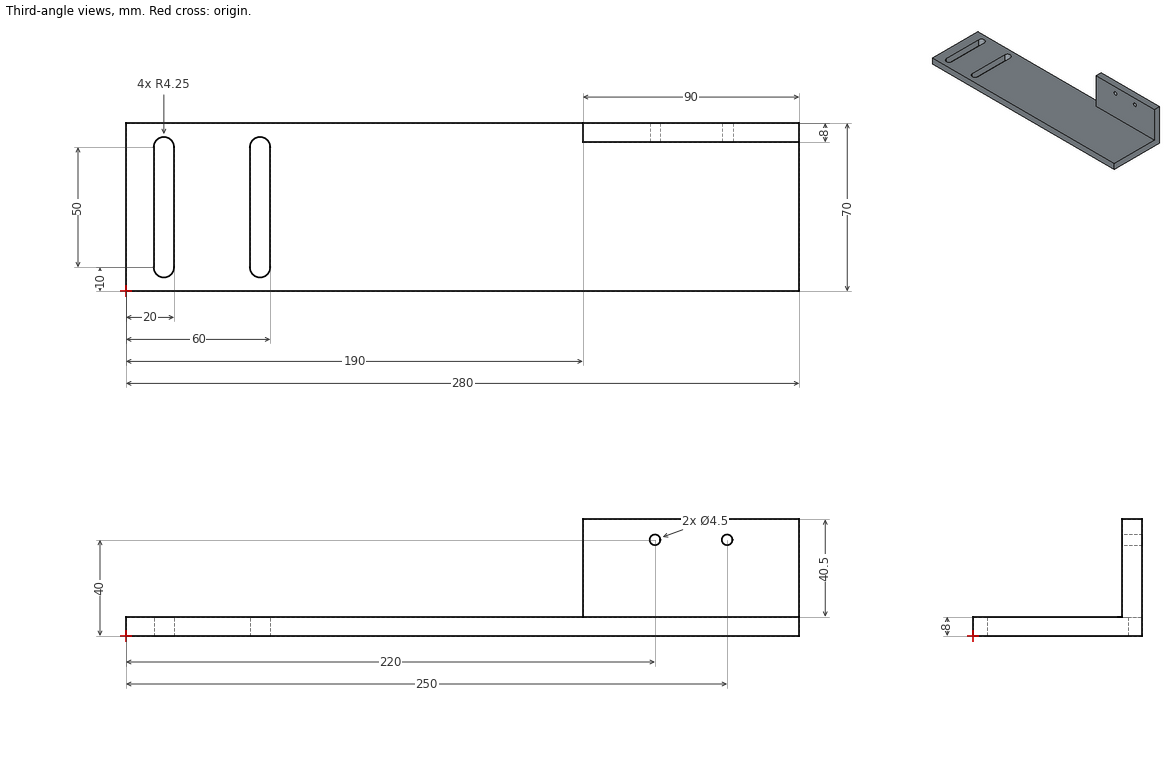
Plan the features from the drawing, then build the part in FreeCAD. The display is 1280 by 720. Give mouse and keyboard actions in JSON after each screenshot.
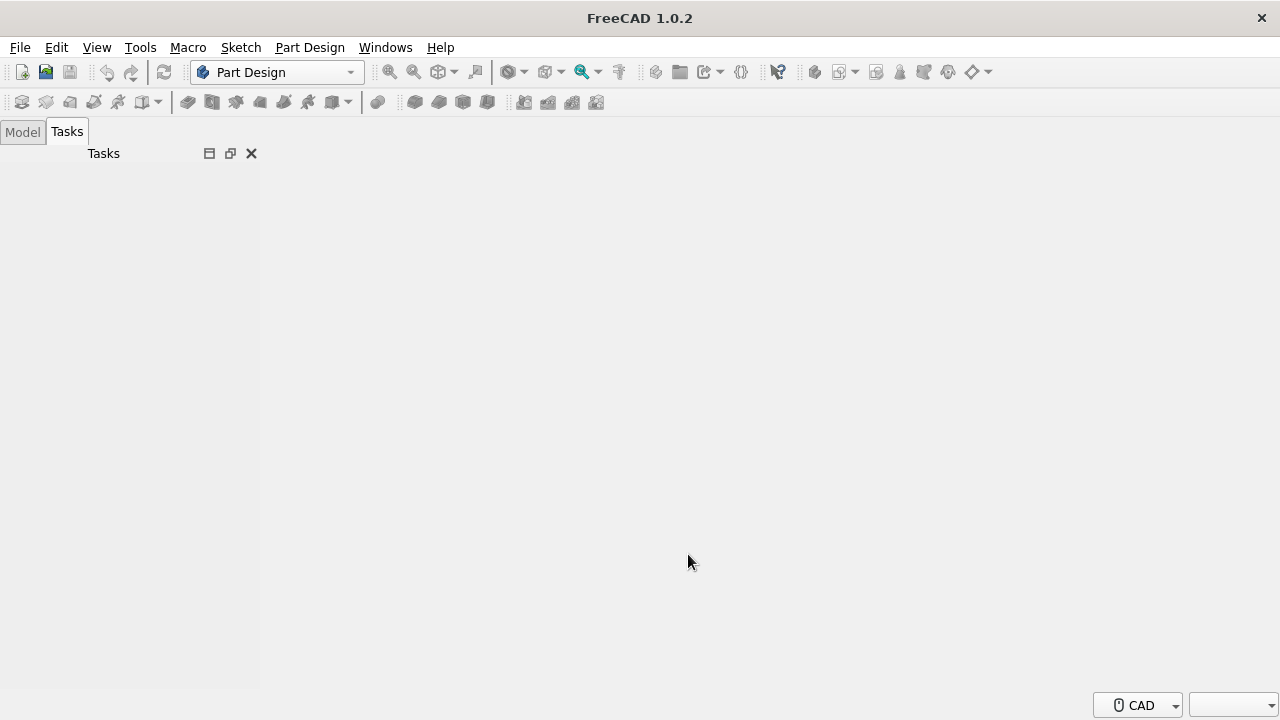
{"action": "key", "text": "ctrl+n"}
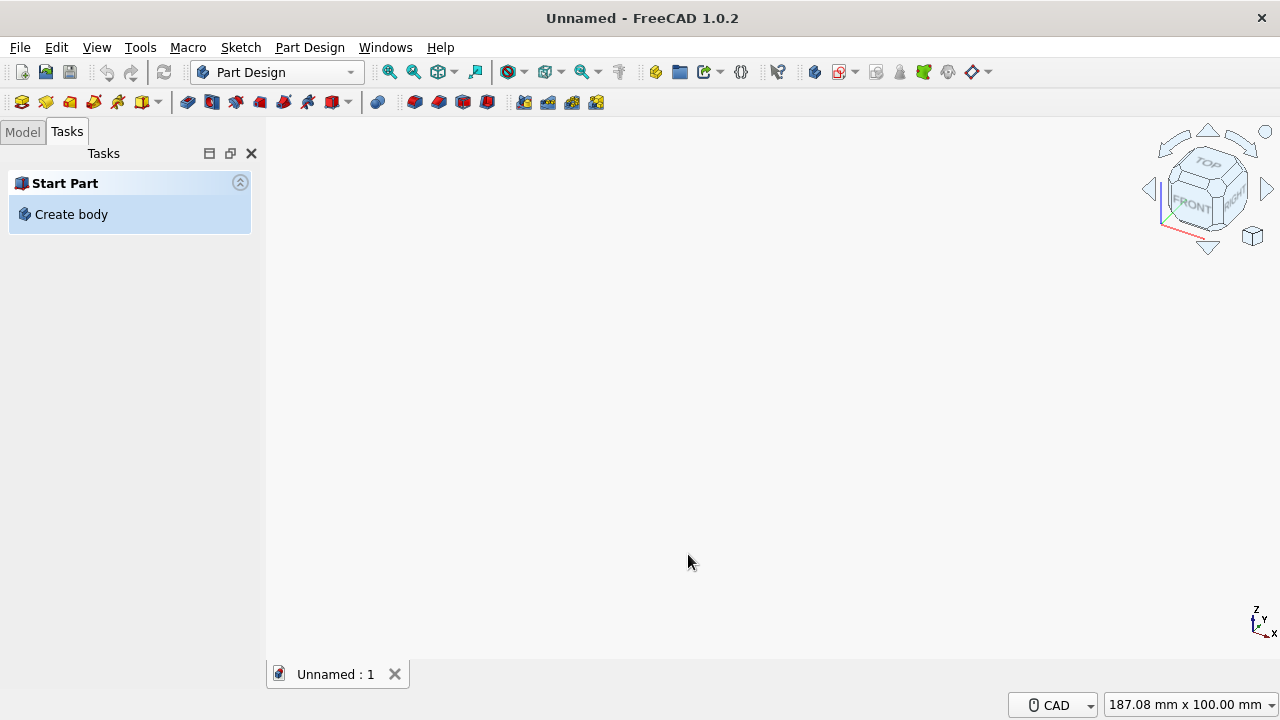
{"action": "left_click", "coordinate": [840, 72]}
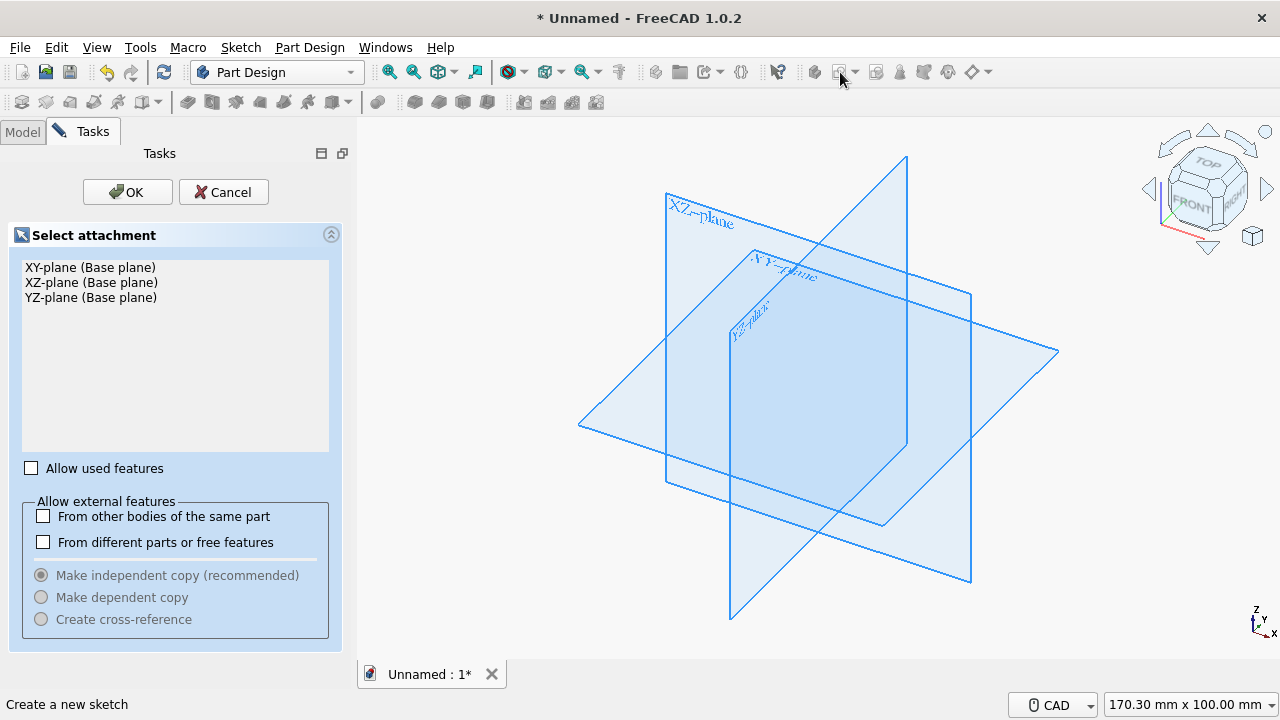
{"action": "left_click", "coordinate": [82, 268]}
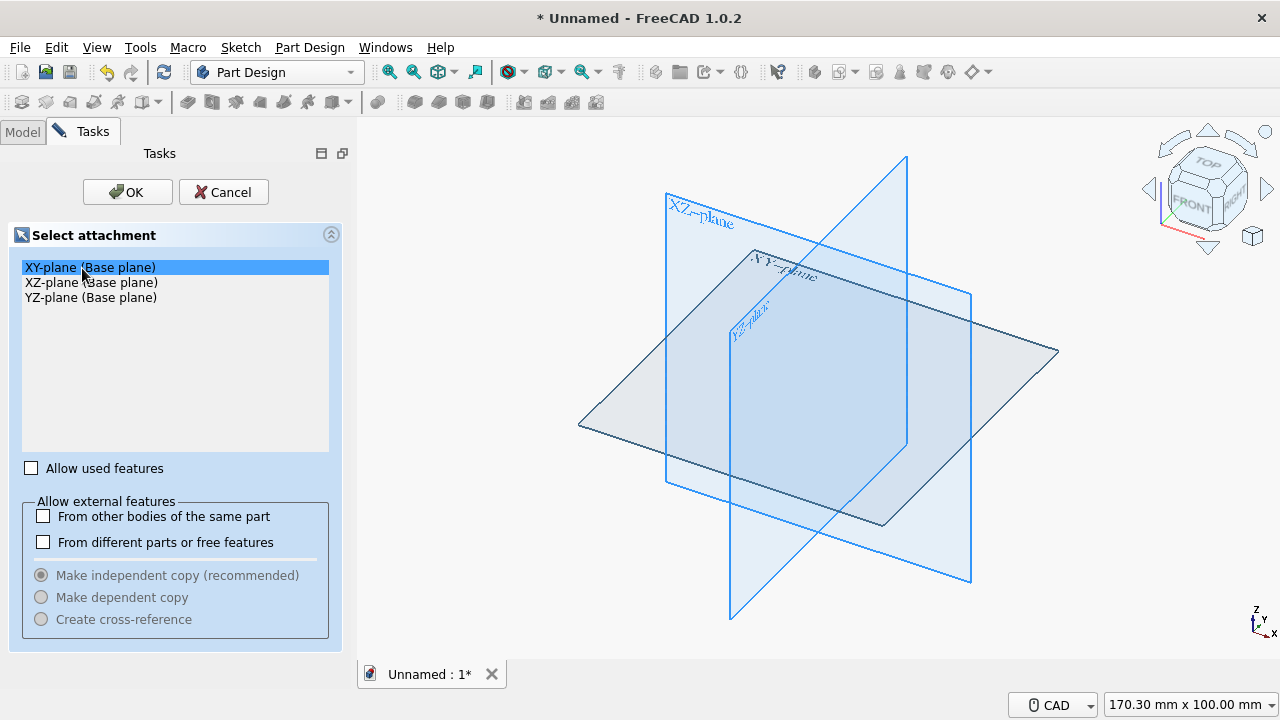
{"action": "left_click", "coordinate": [128, 192]}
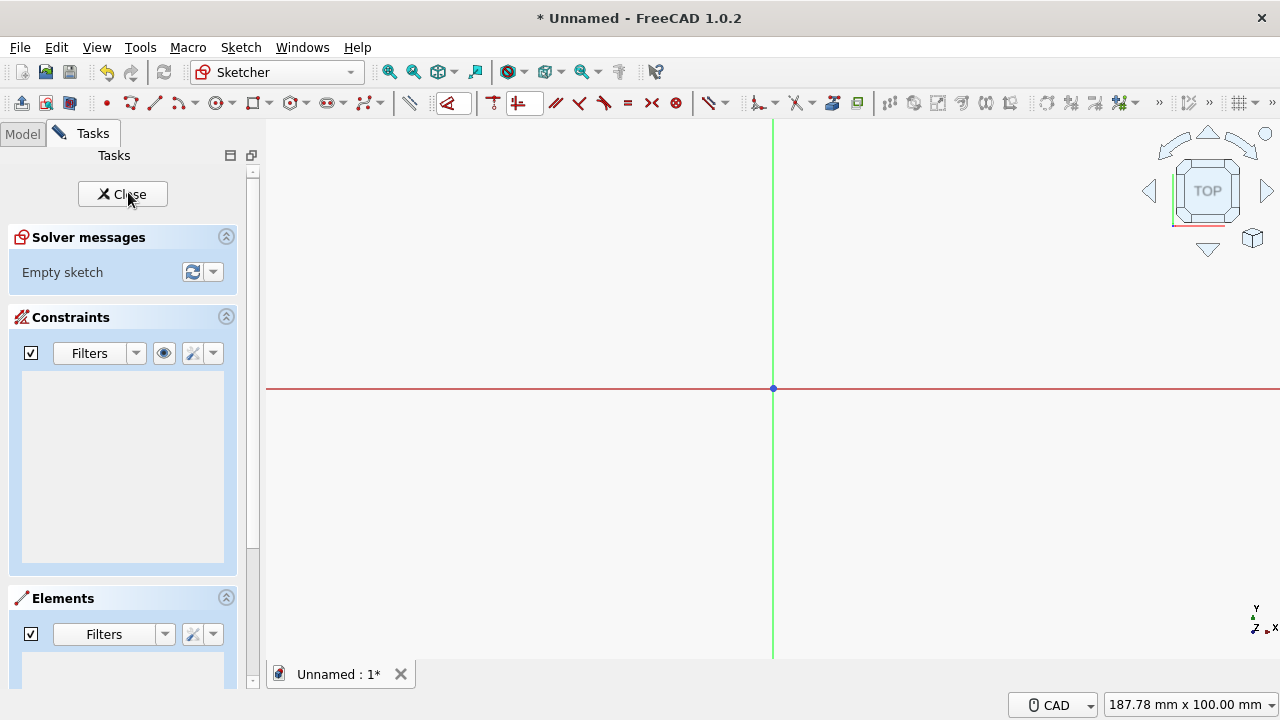
{"action": "scroll", "coordinate": [294, 499], "scroll_direction": "down", "scroll_amount": 5}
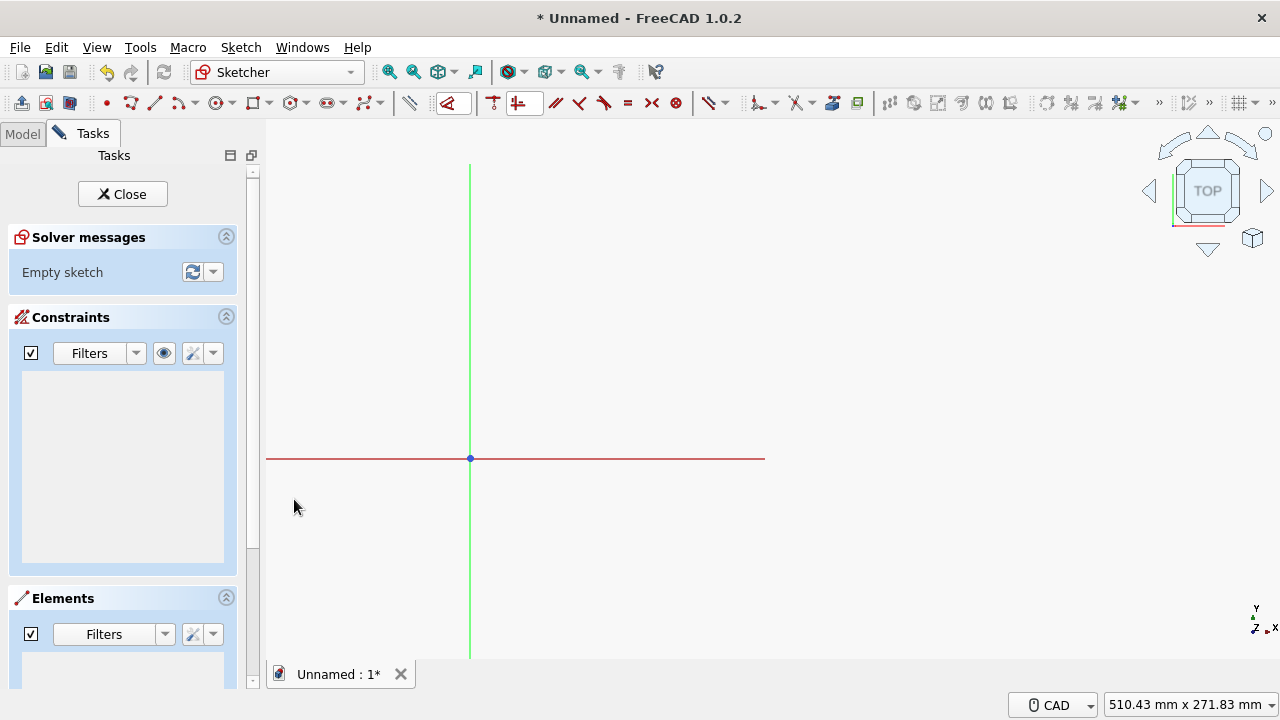
{"action": "left_click", "coordinate": [254, 104]}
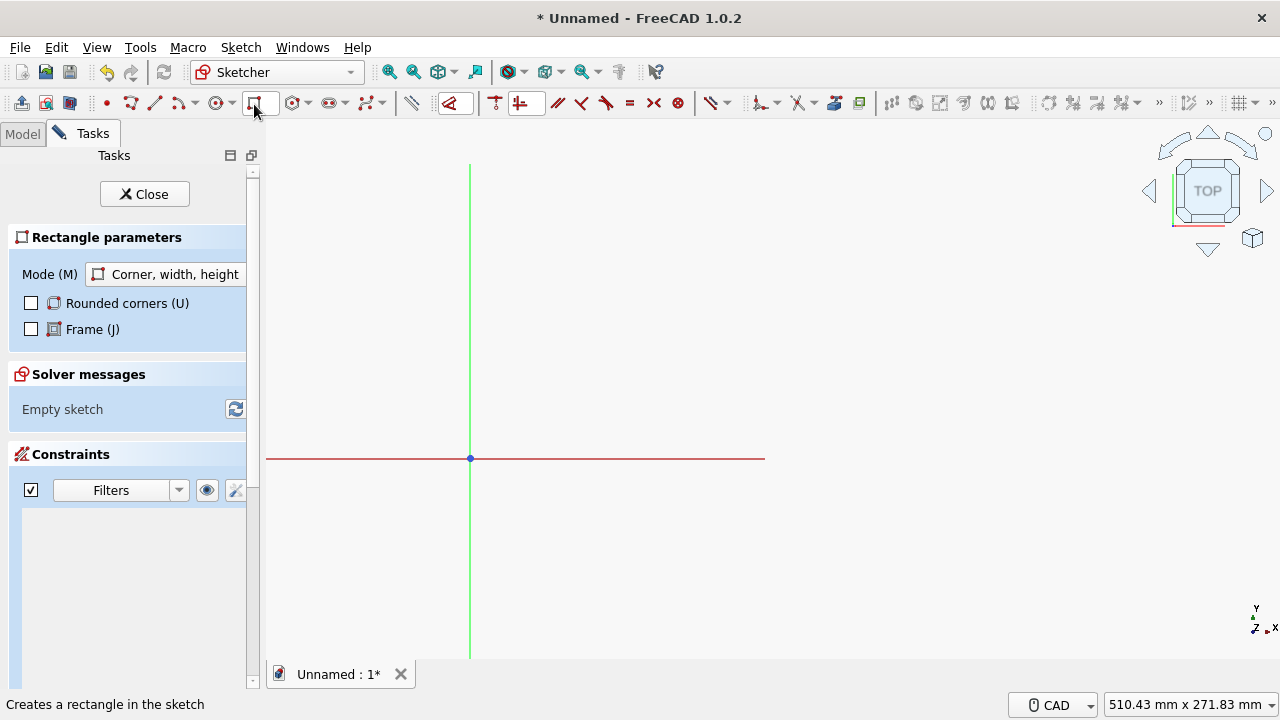
{"action": "left_click", "coordinate": [470, 459]}
{"action": "mouse_move", "coordinate": [1026, 320]}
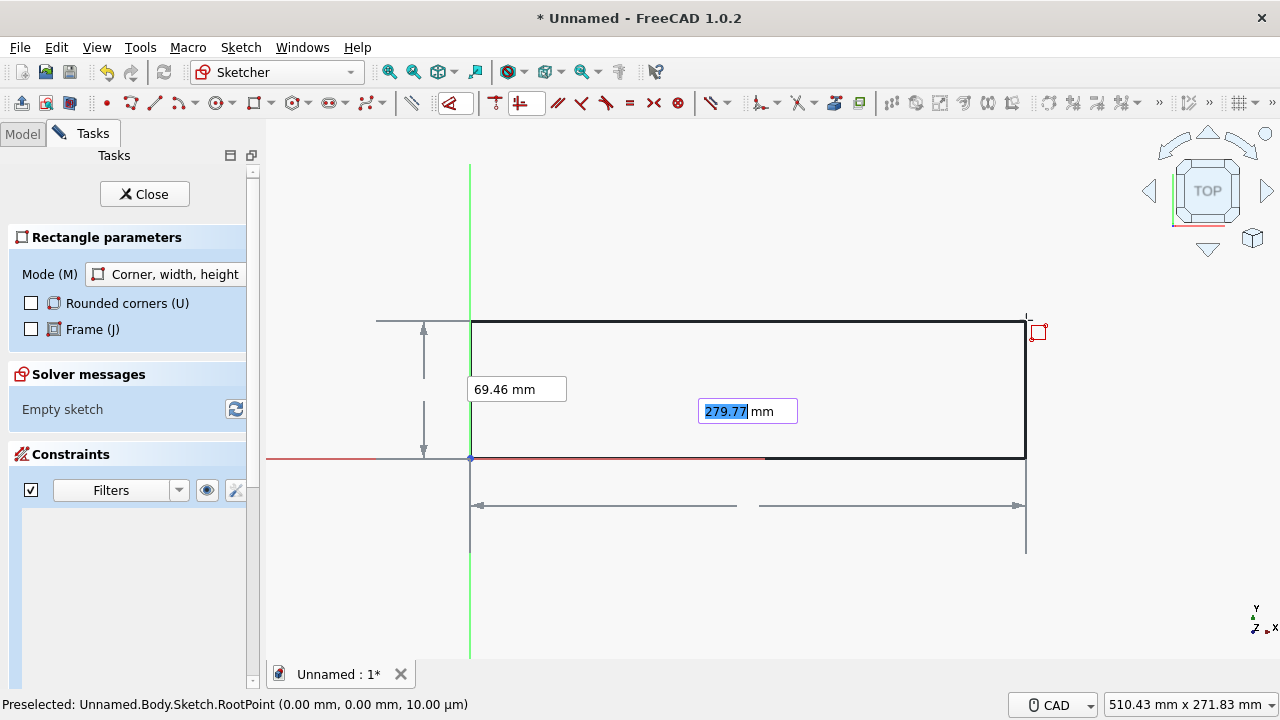
{"action": "type", "text": "280"}
{"action": "key", "text": "Tab"}
{"action": "type", "text": "70"}
{"action": "key", "text": "Return"}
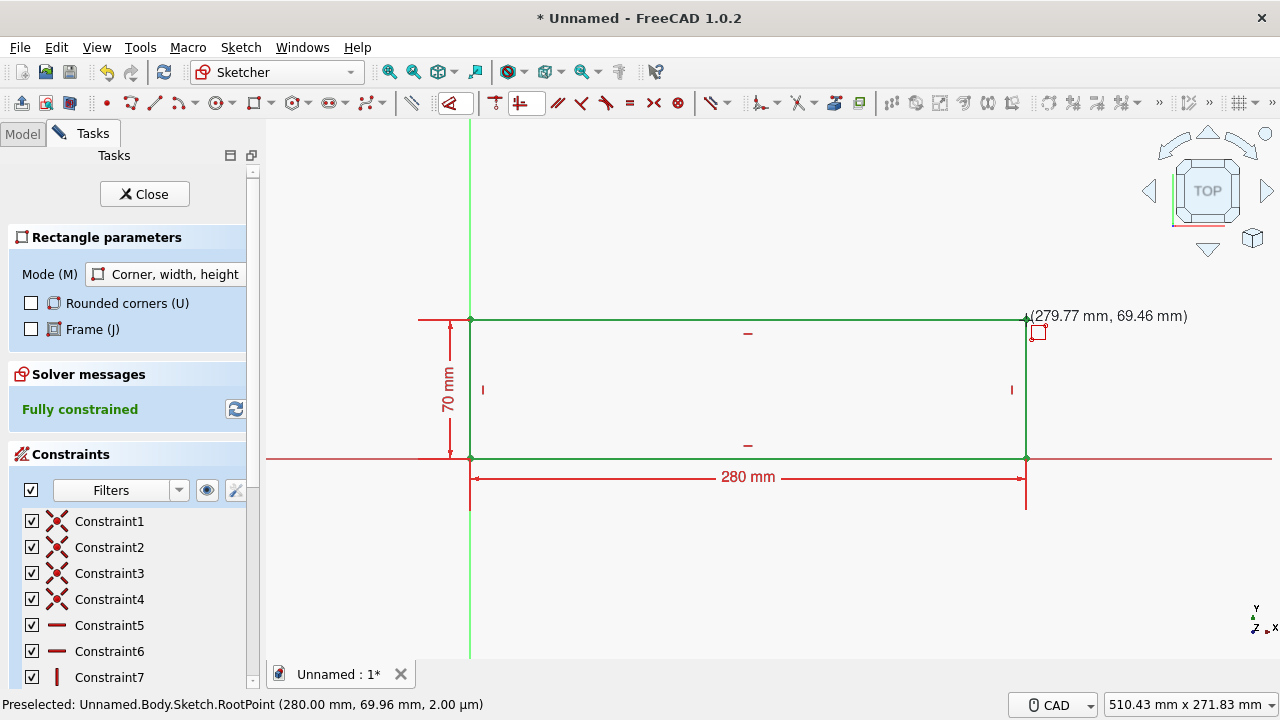
{"action": "key", "text": "g s"}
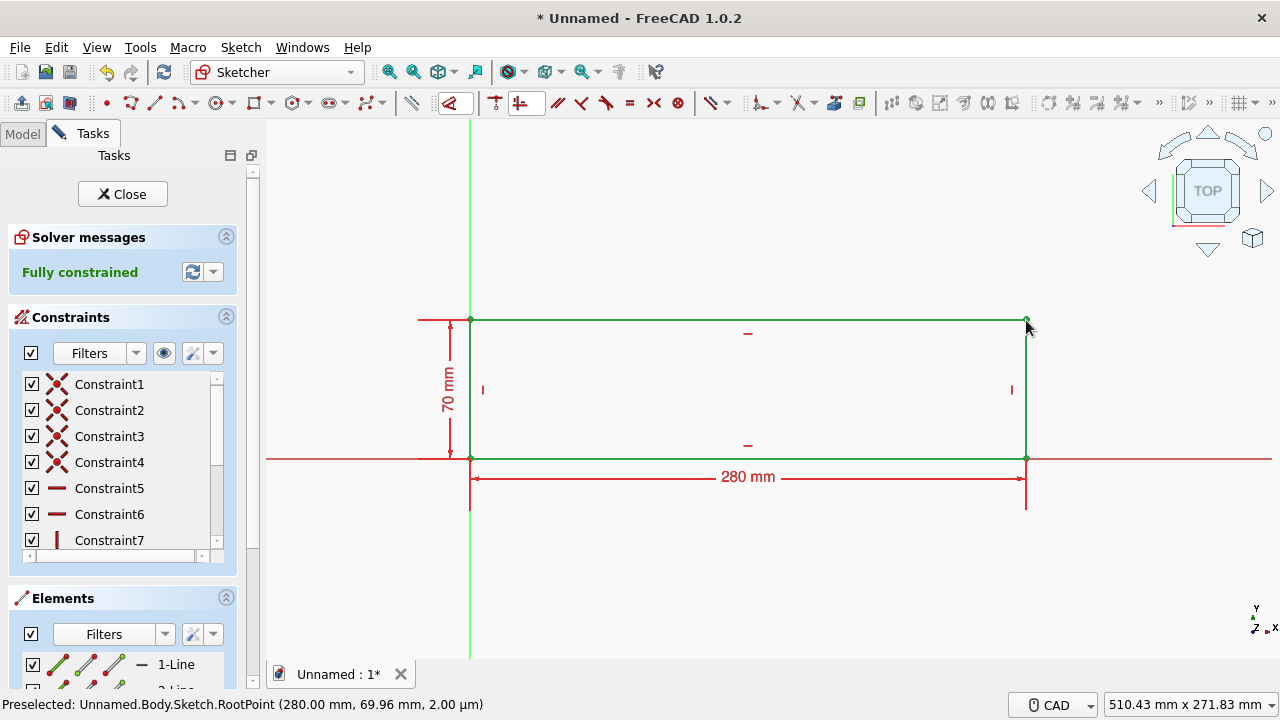
{"action": "scroll", "coordinate": [502, 439], "scroll_direction": "up", "scroll_amount": 5}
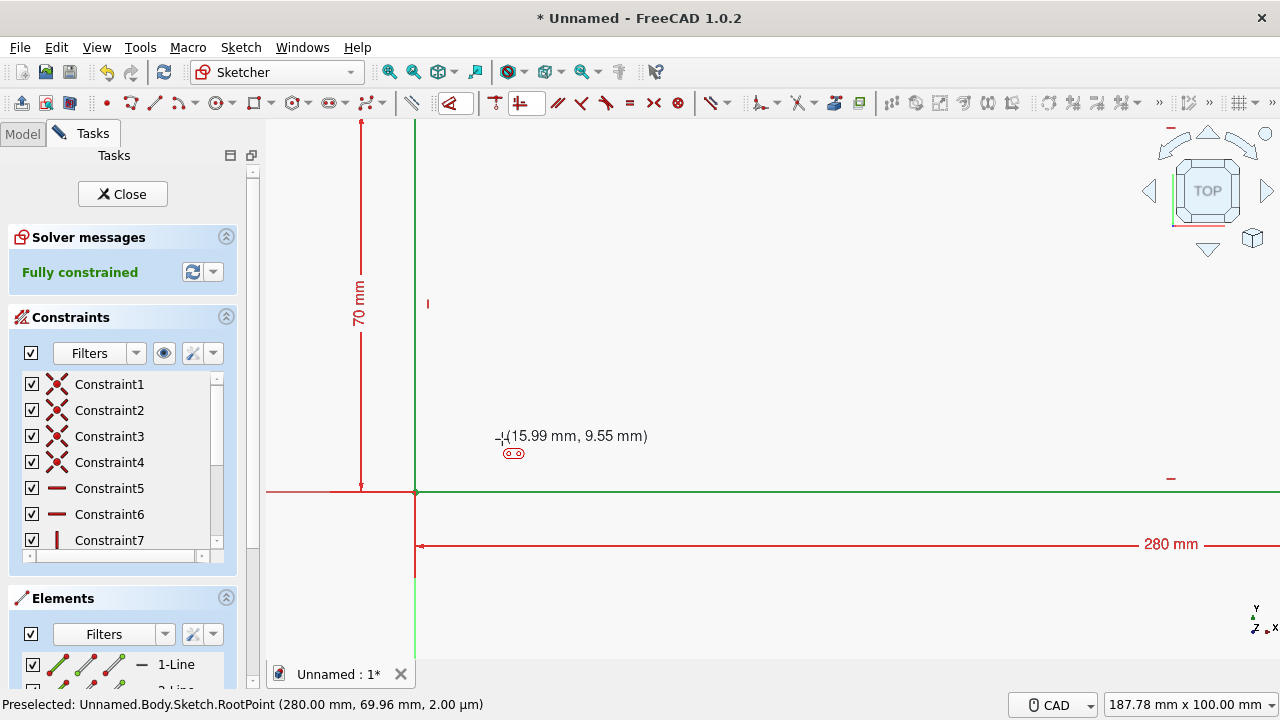
{"action": "left_click", "coordinate": [500, 438]}